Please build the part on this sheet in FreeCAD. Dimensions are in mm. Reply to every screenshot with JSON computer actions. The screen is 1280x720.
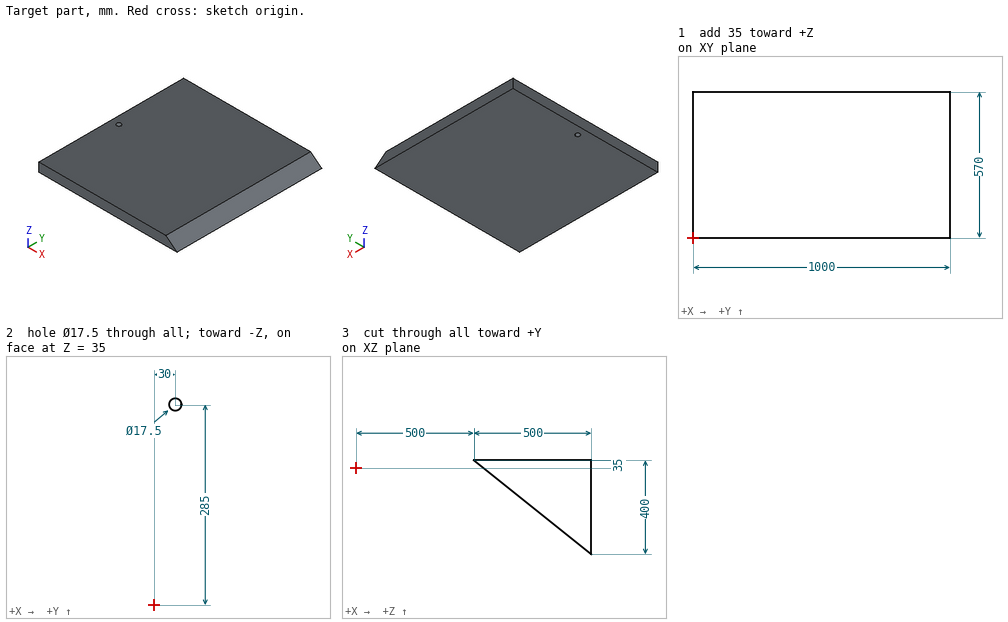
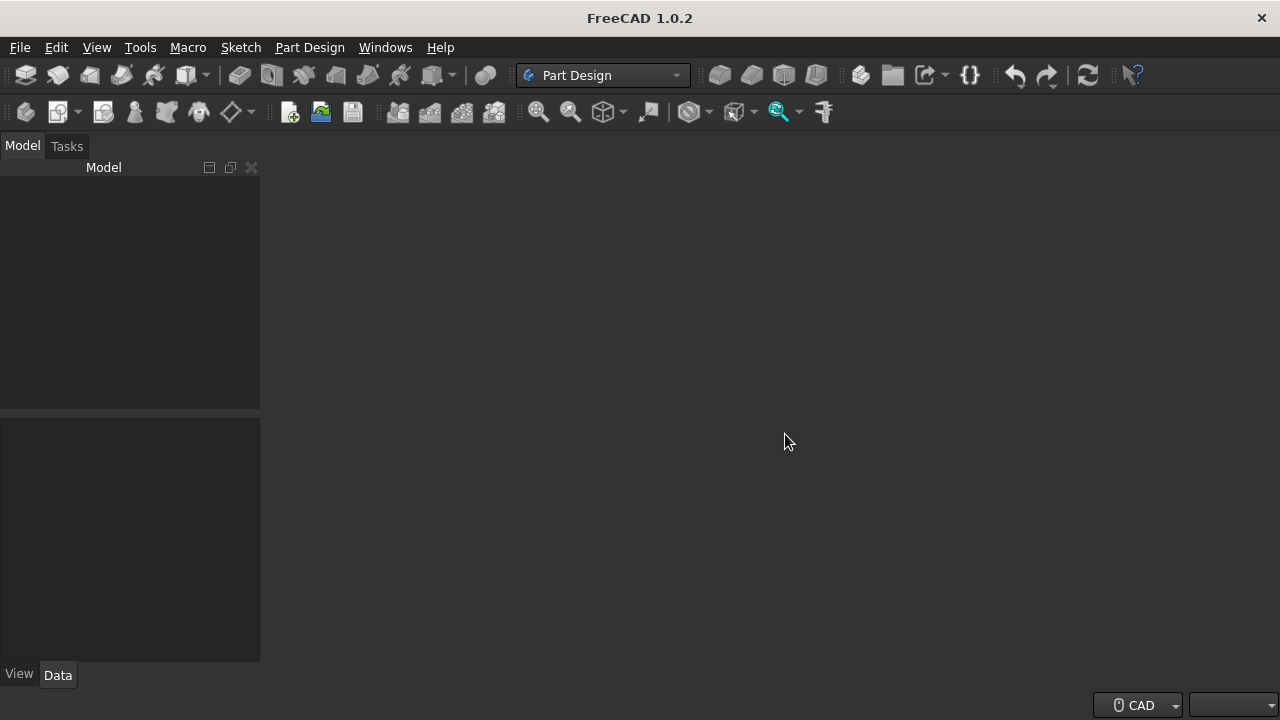
{"action": "left_click", "coordinate": [290, 112]}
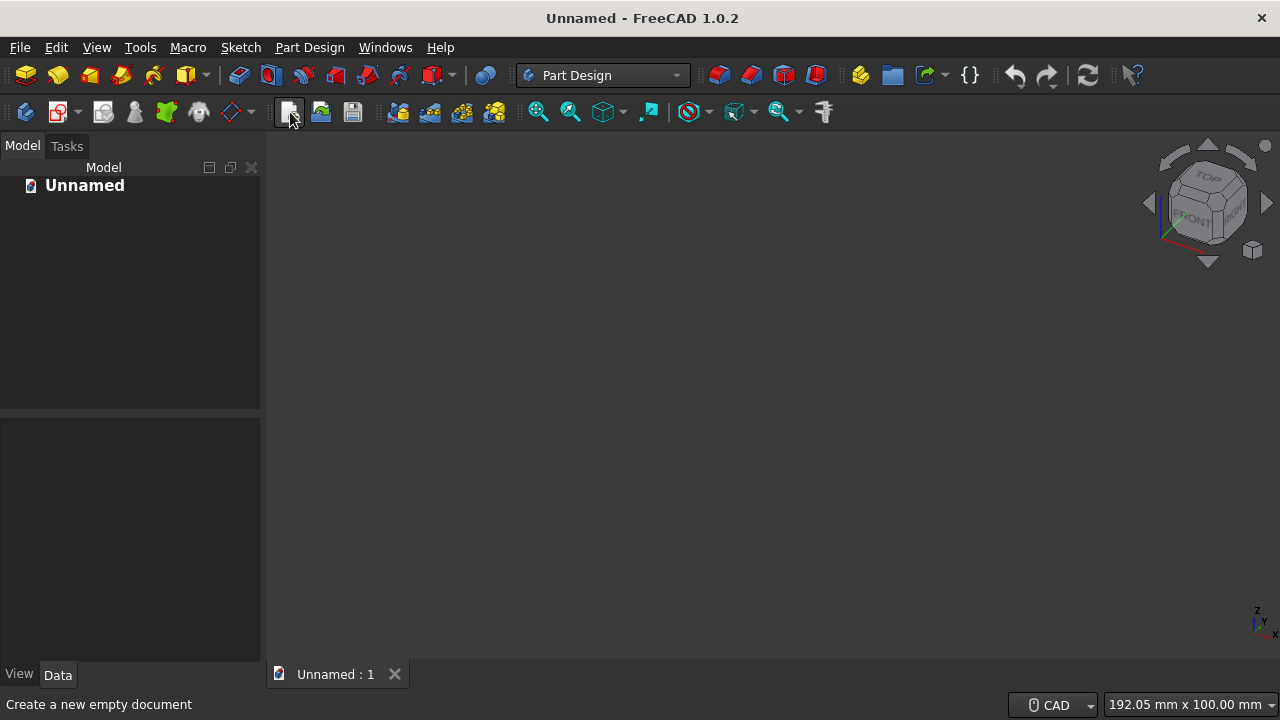
{"action": "left_click", "coordinate": [58, 112]}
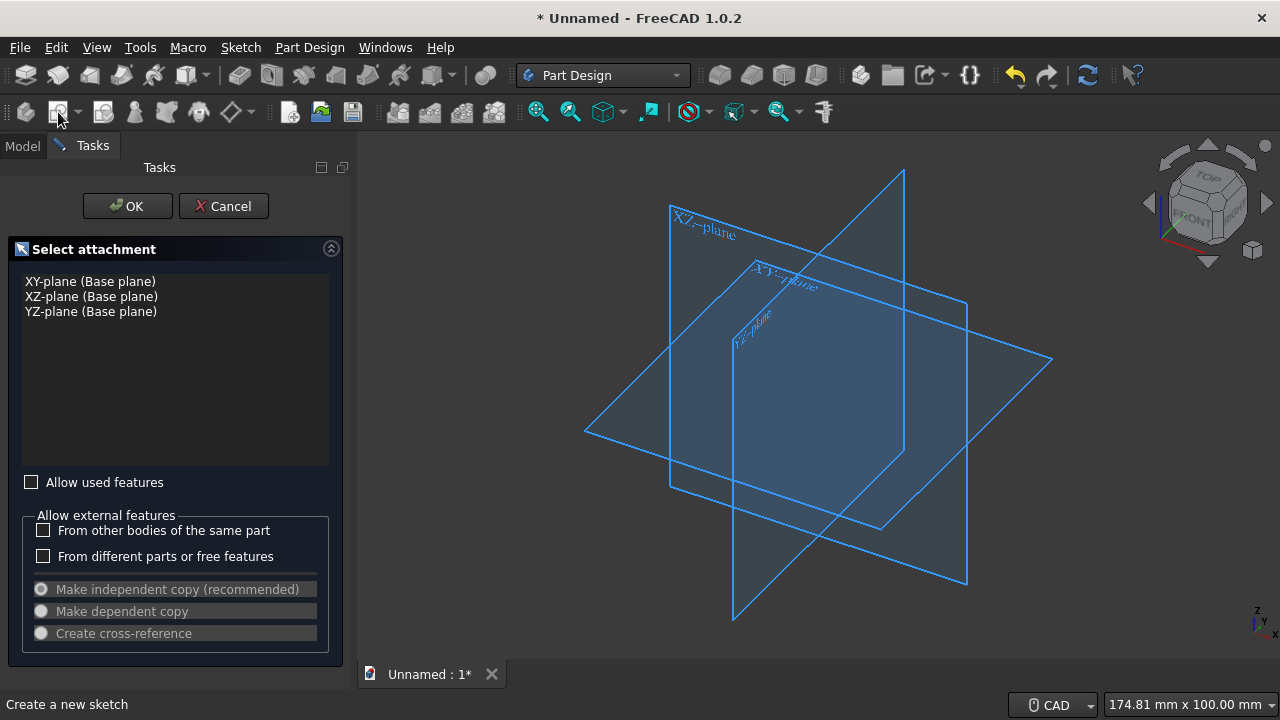
{"action": "left_click", "coordinate": [82, 282]}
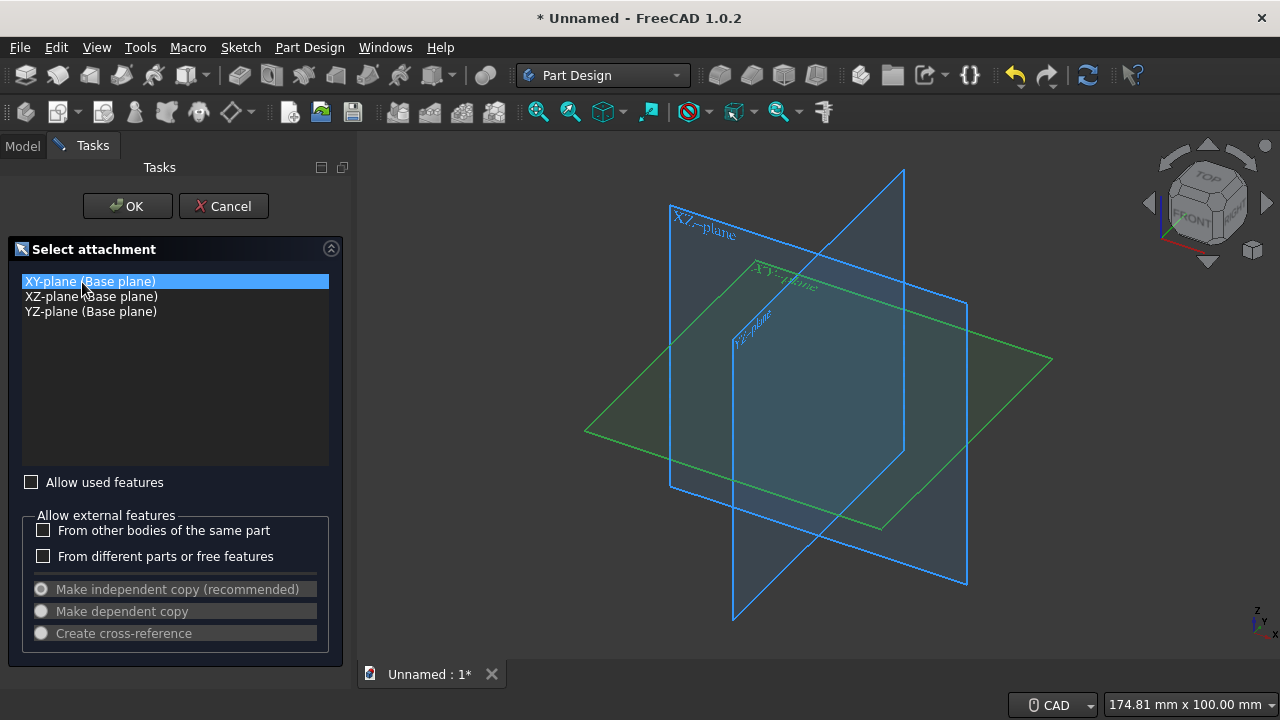
{"action": "left_click", "coordinate": [128, 206]}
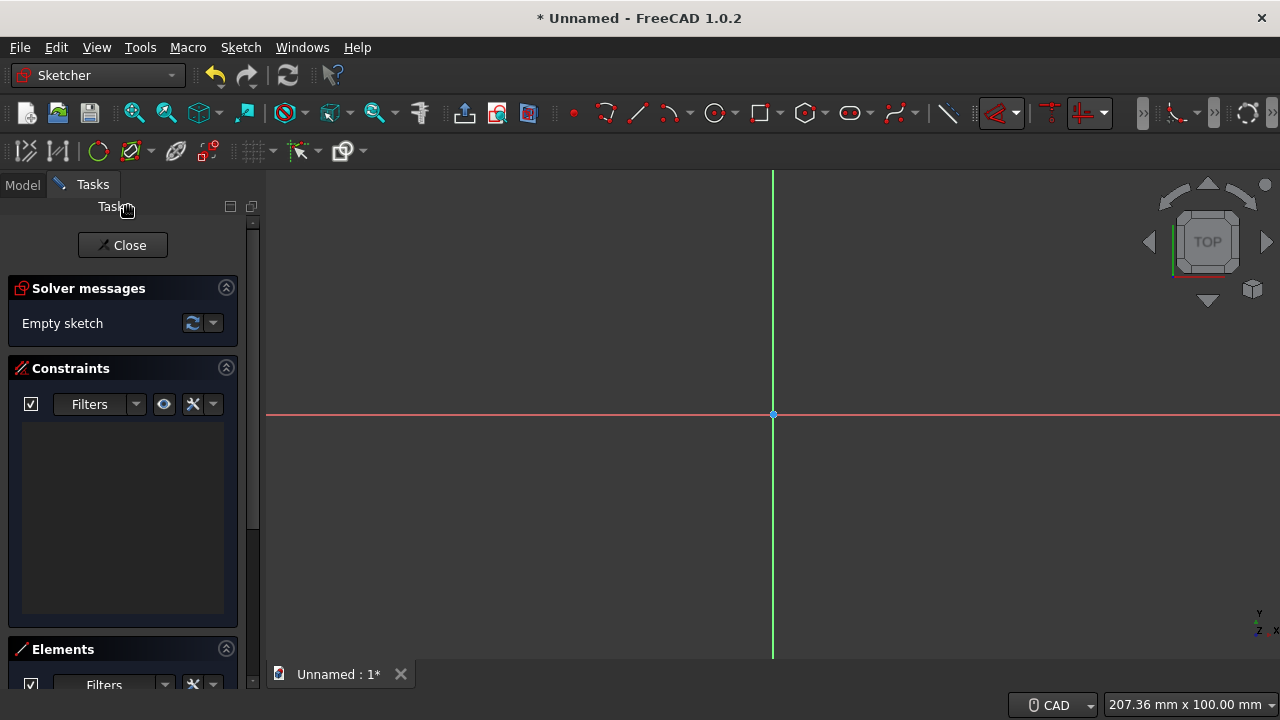
{"action": "scroll", "coordinate": [391, 588], "scroll_direction": "down", "scroll_amount": 11}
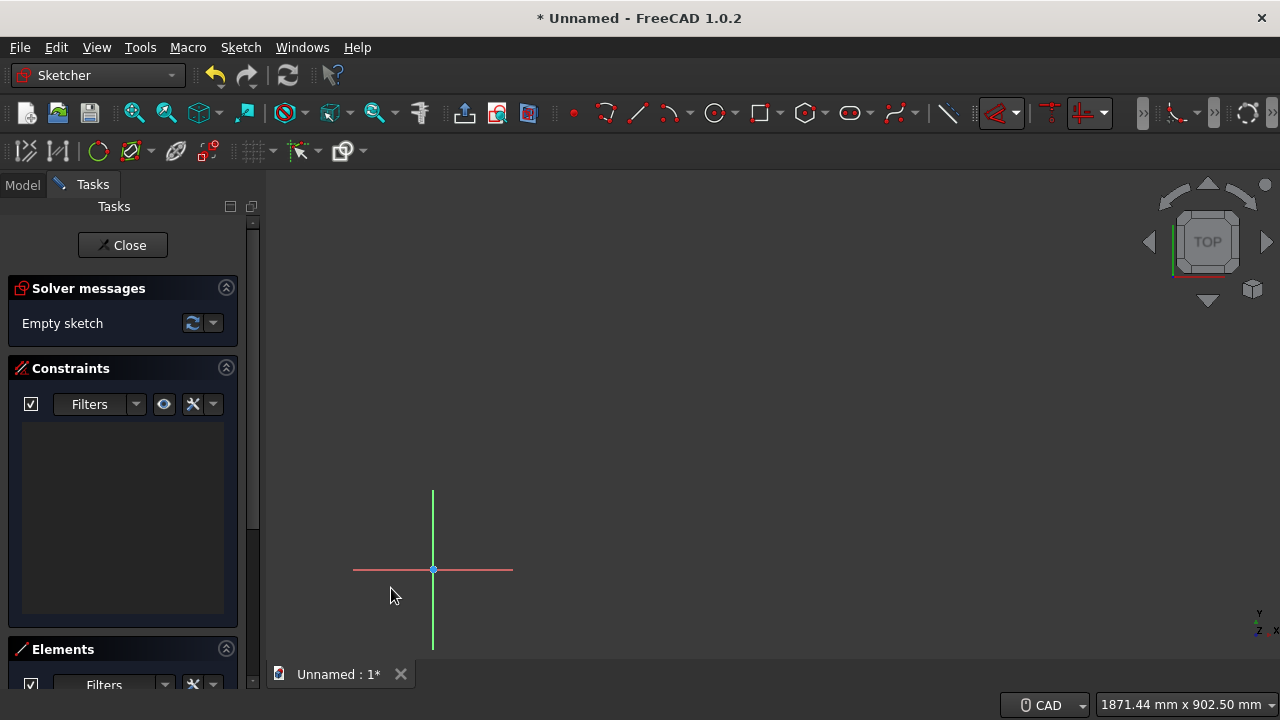
{"action": "left_click", "coordinate": [760, 114]}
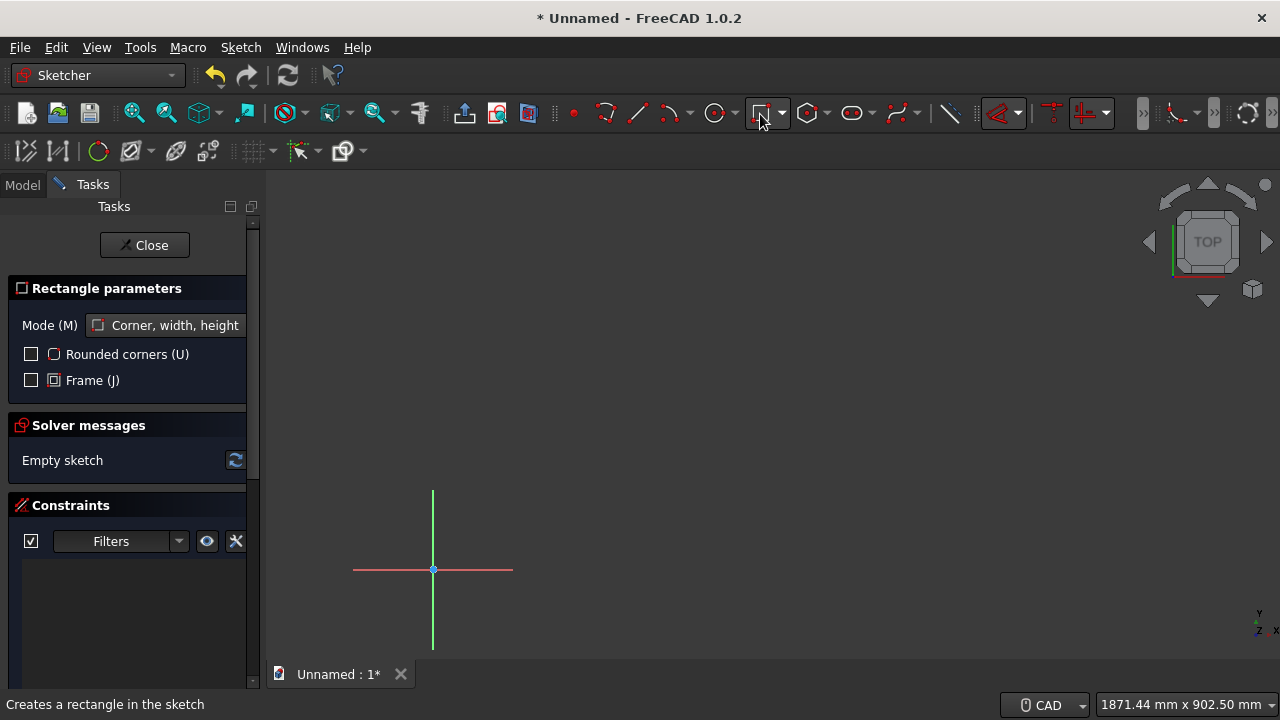
{"action": "left_click", "coordinate": [433, 570]}
{"action": "mouse_move", "coordinate": [975, 261]}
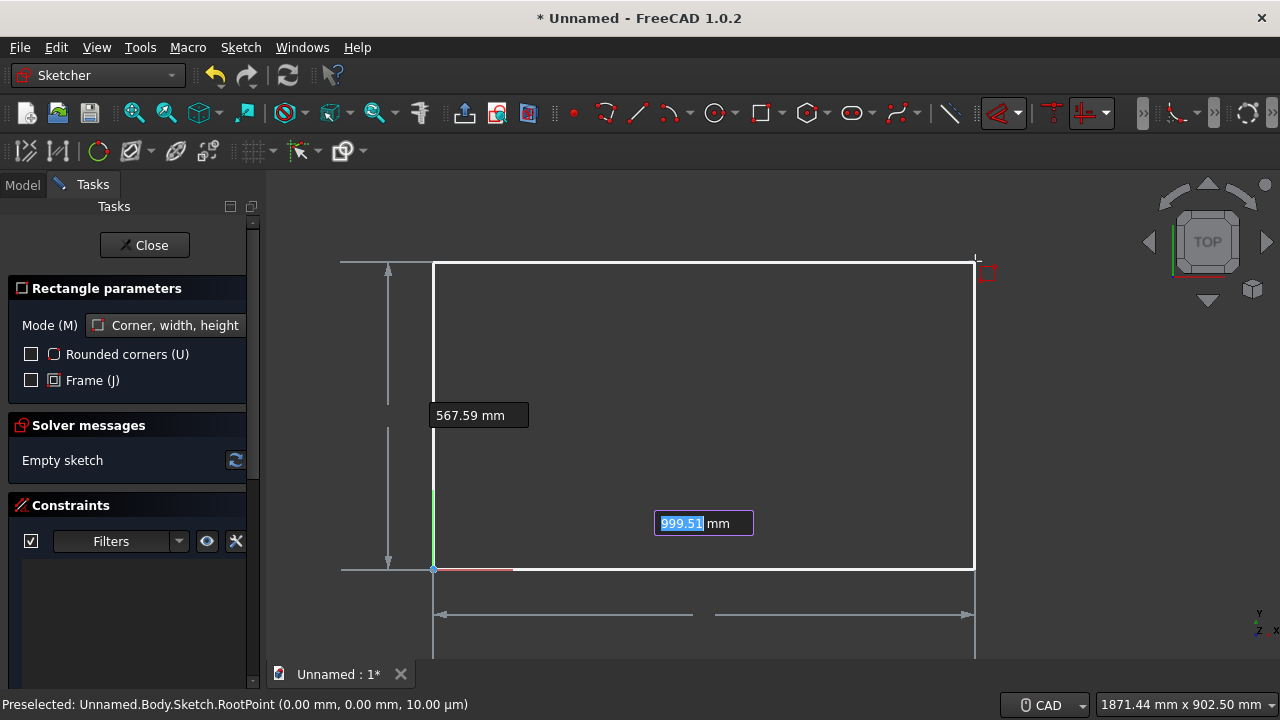
{"action": "type", "text": "1000"}
{"action": "key", "text": "Tab"}
{"action": "type", "text": "570"}
{"action": "key", "text": "Return"}
{"action": "key", "text": "Escape"}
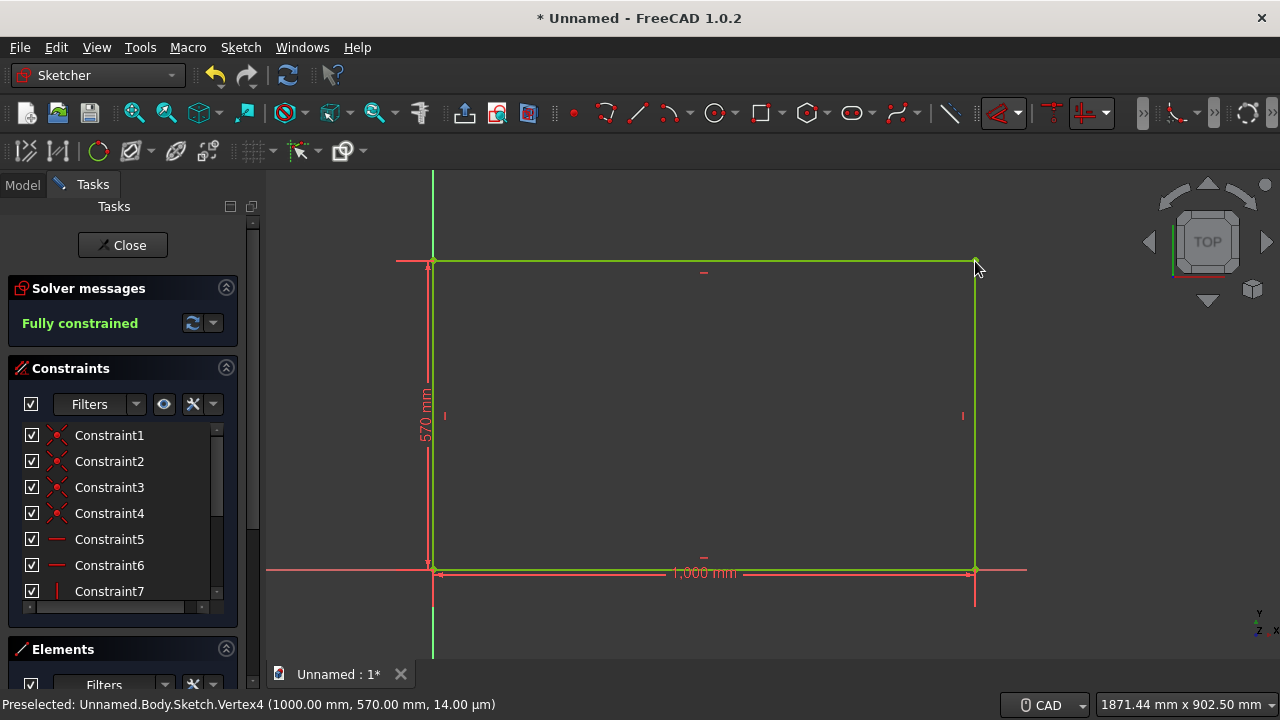
{"action": "left_click", "coordinate": [123, 245]}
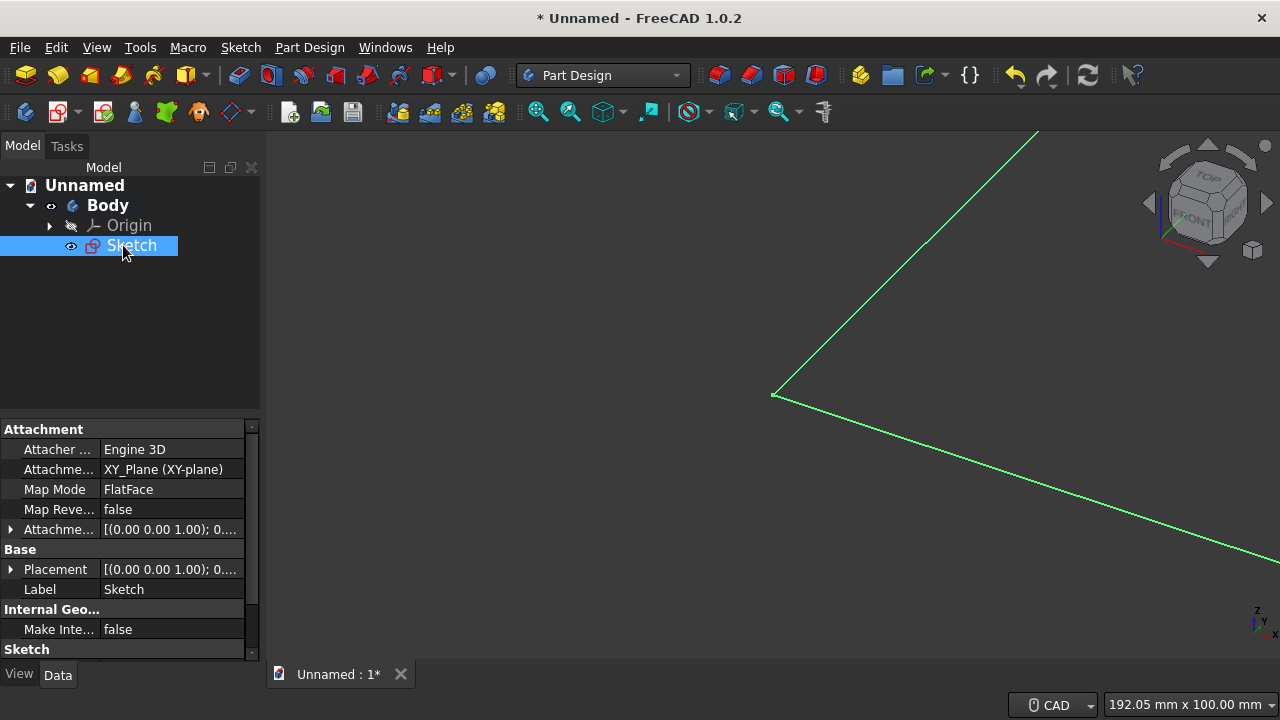
{"action": "left_click", "coordinate": [26, 76]}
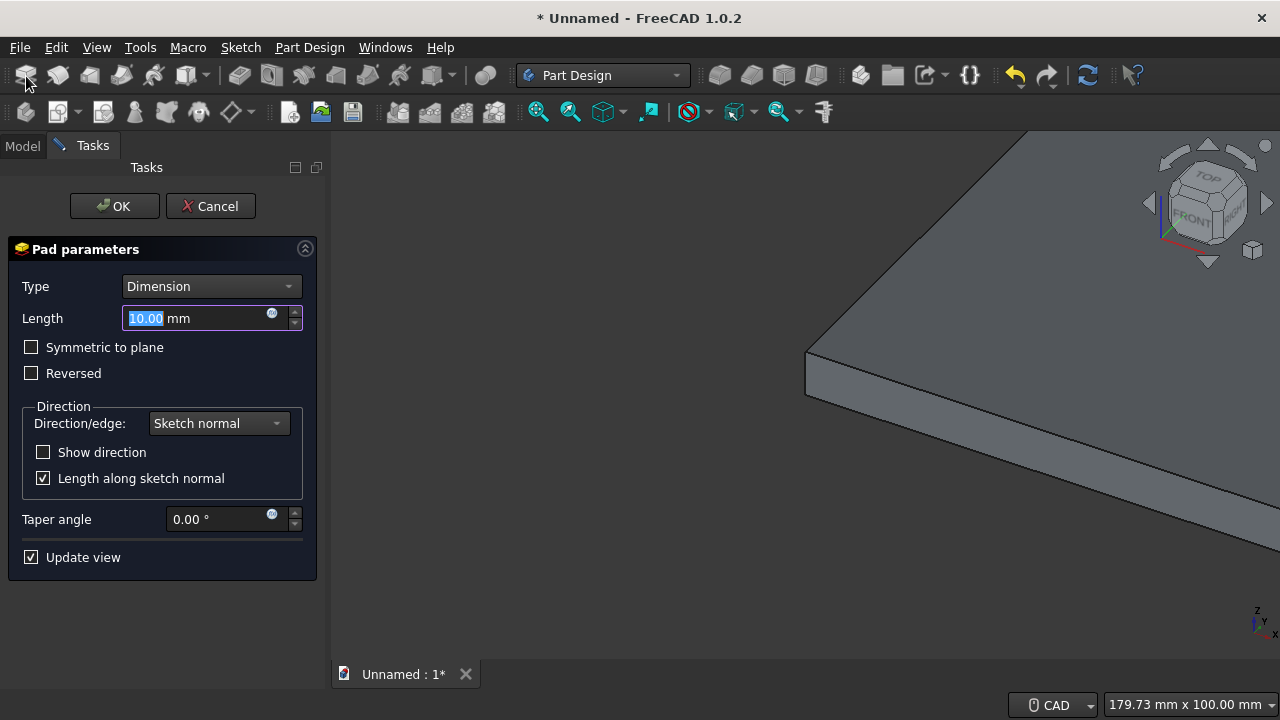
{"action": "type", "text": "35"}
{"action": "key", "text": "Tab"}